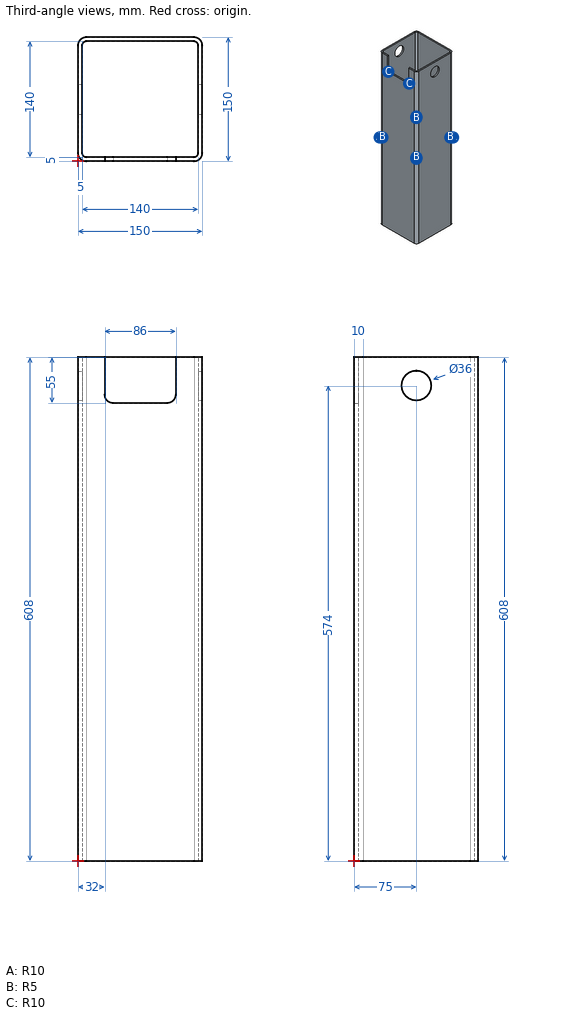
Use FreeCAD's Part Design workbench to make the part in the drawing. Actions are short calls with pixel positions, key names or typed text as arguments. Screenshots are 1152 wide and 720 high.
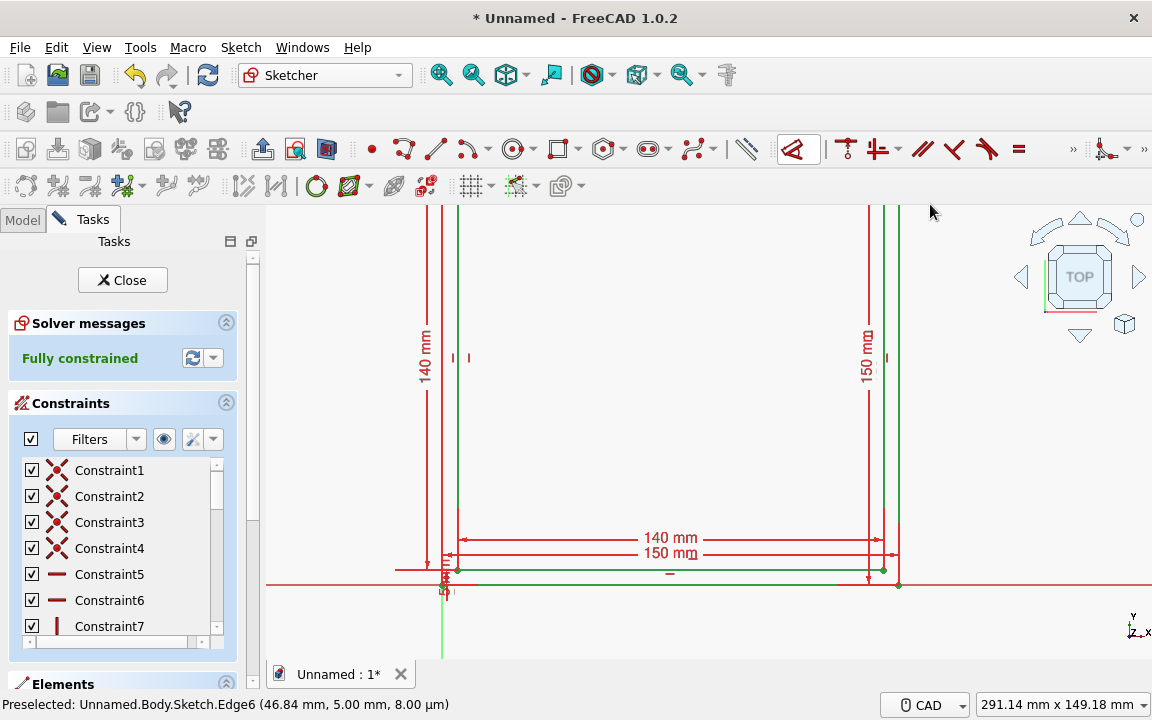
click(123, 280)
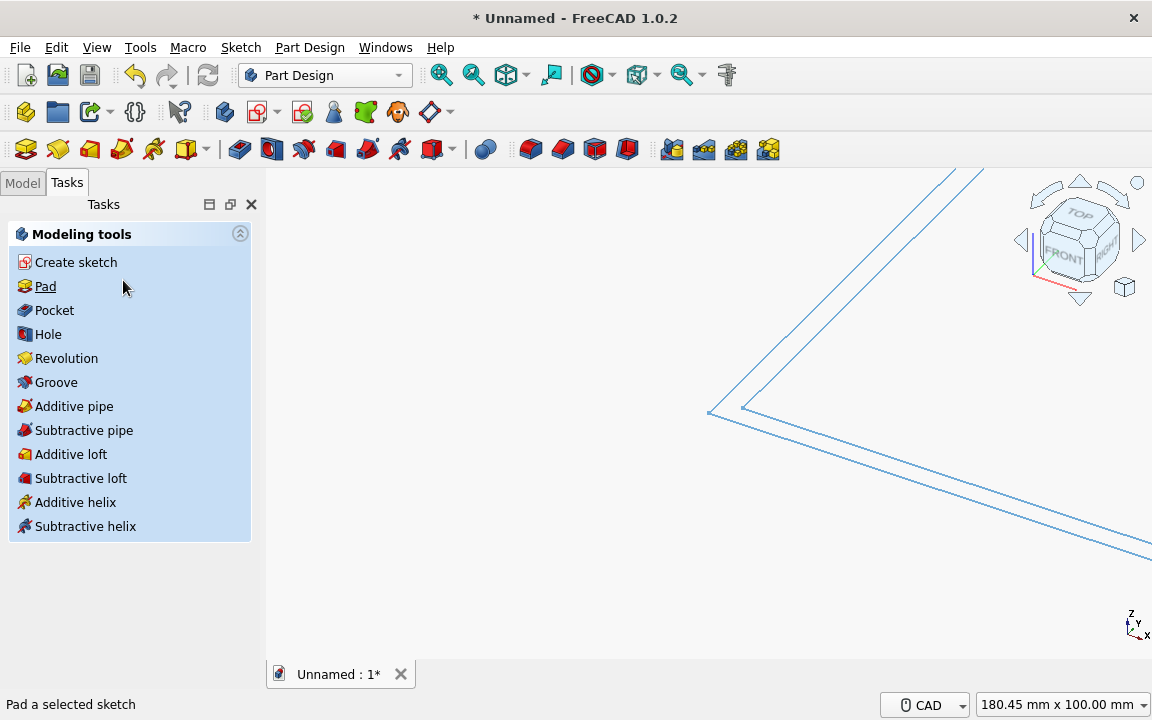
click(26, 150)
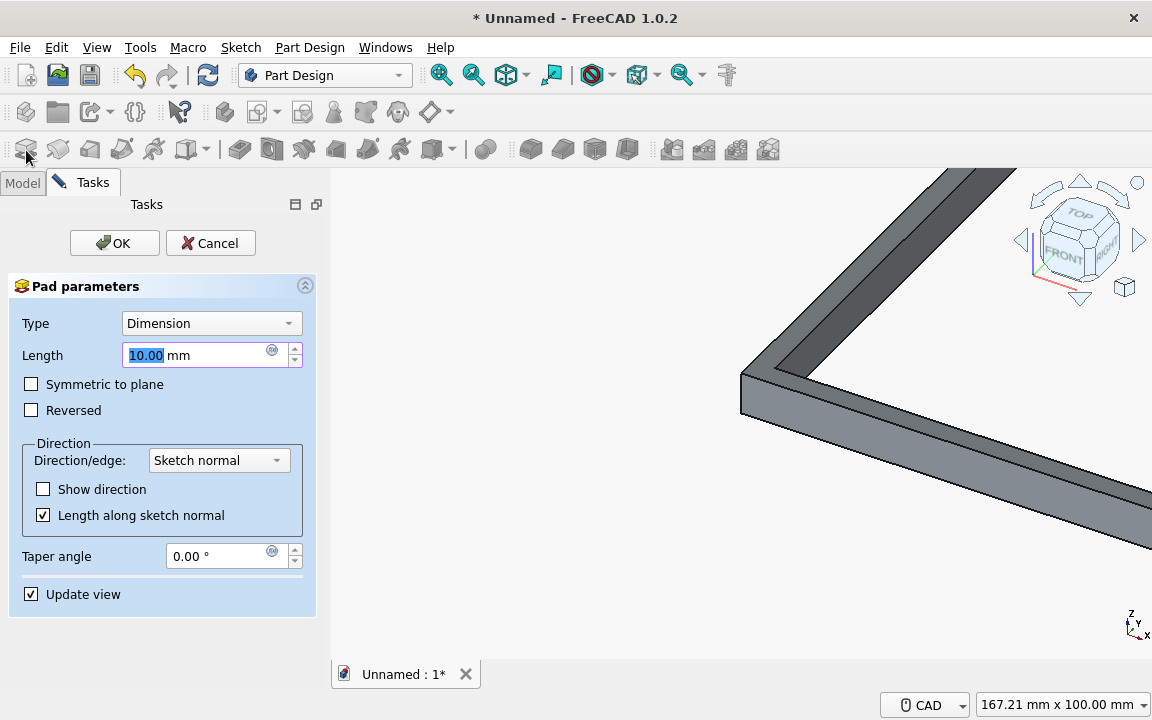
text(608)
key(Tab)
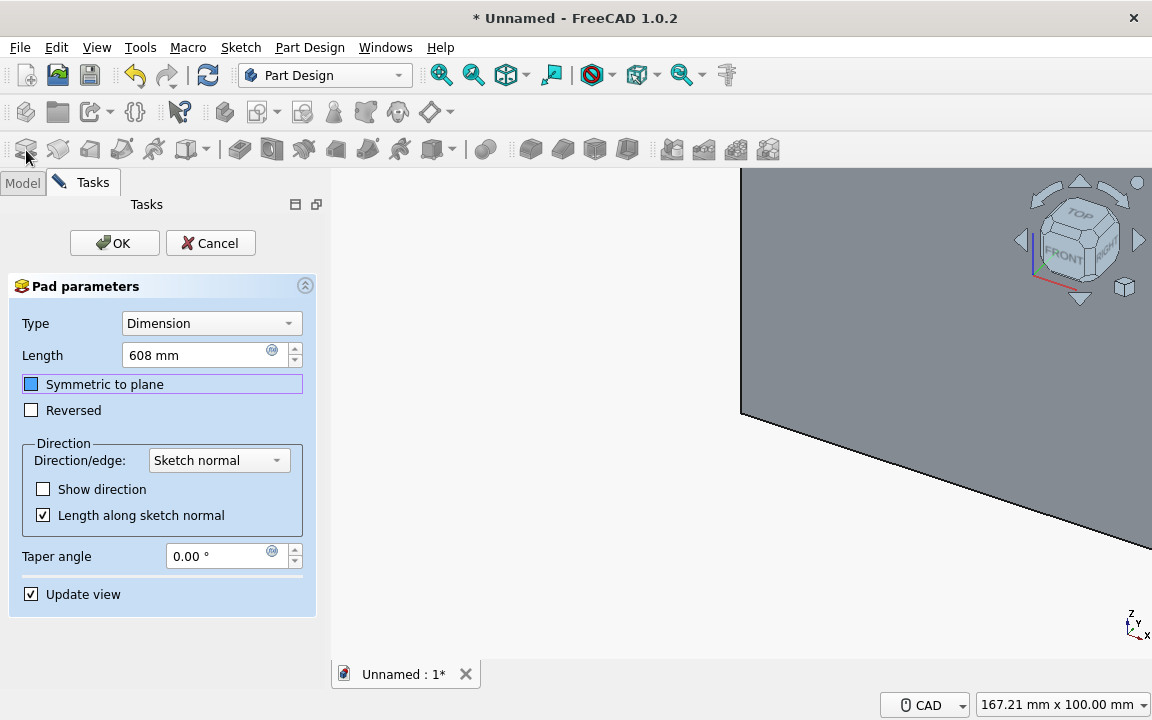
click(115, 243)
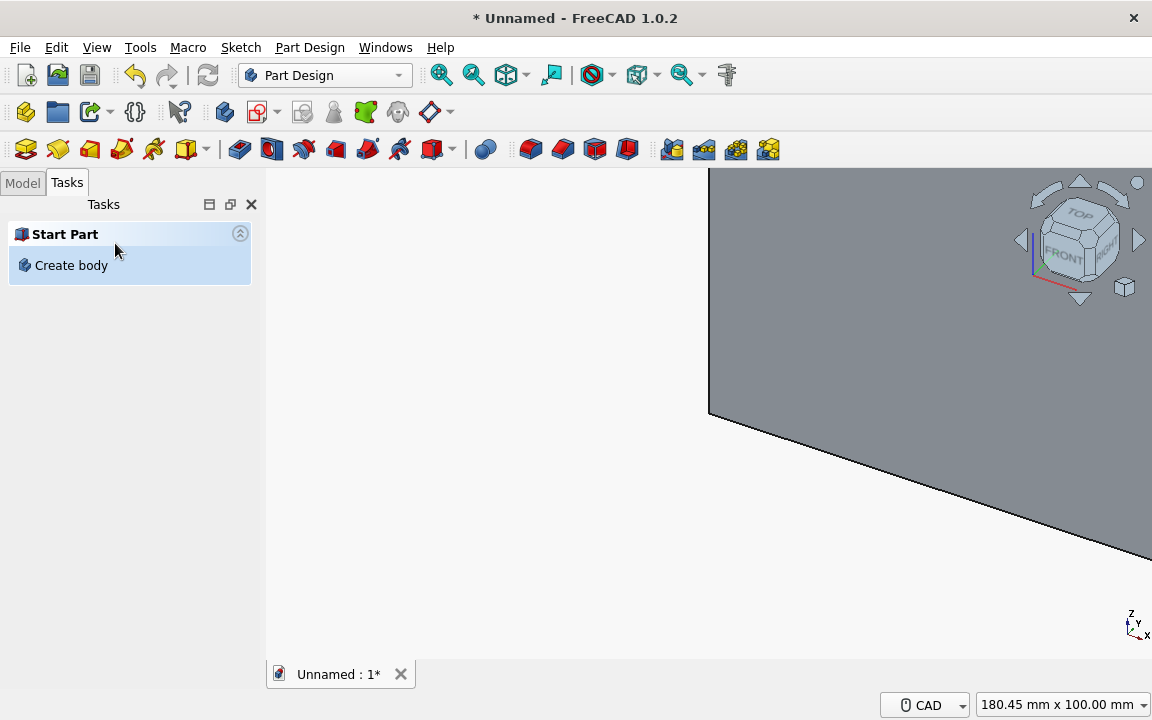
key(v)
key(f)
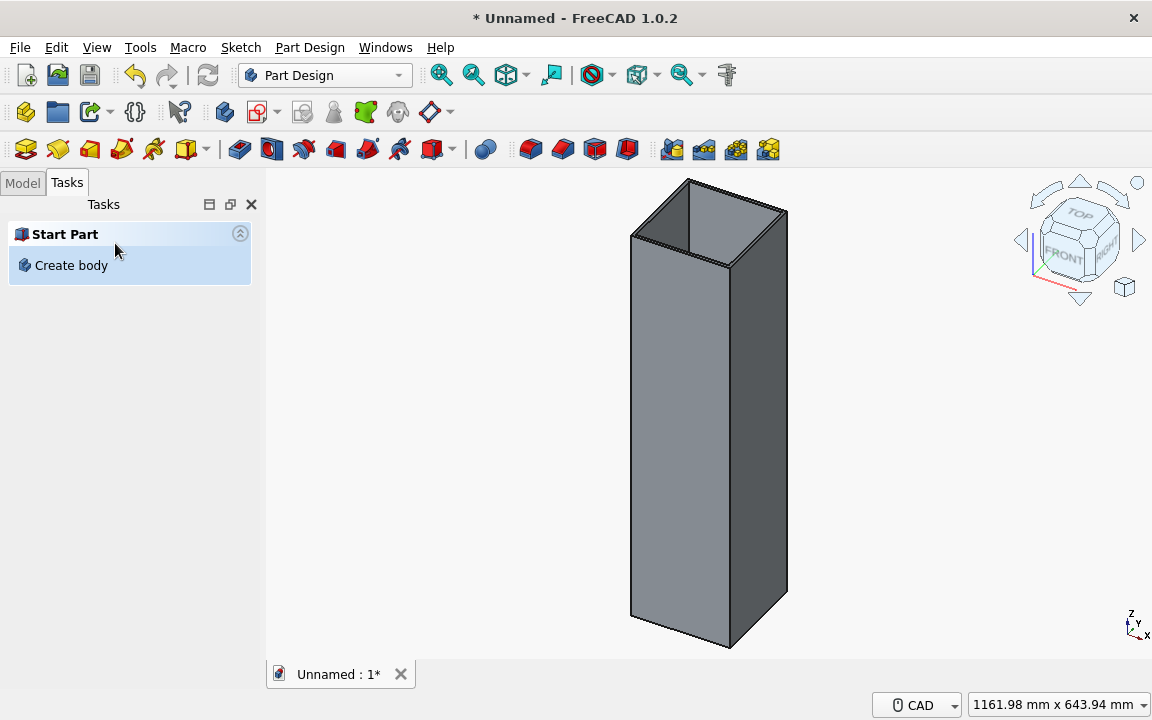
click(730, 457)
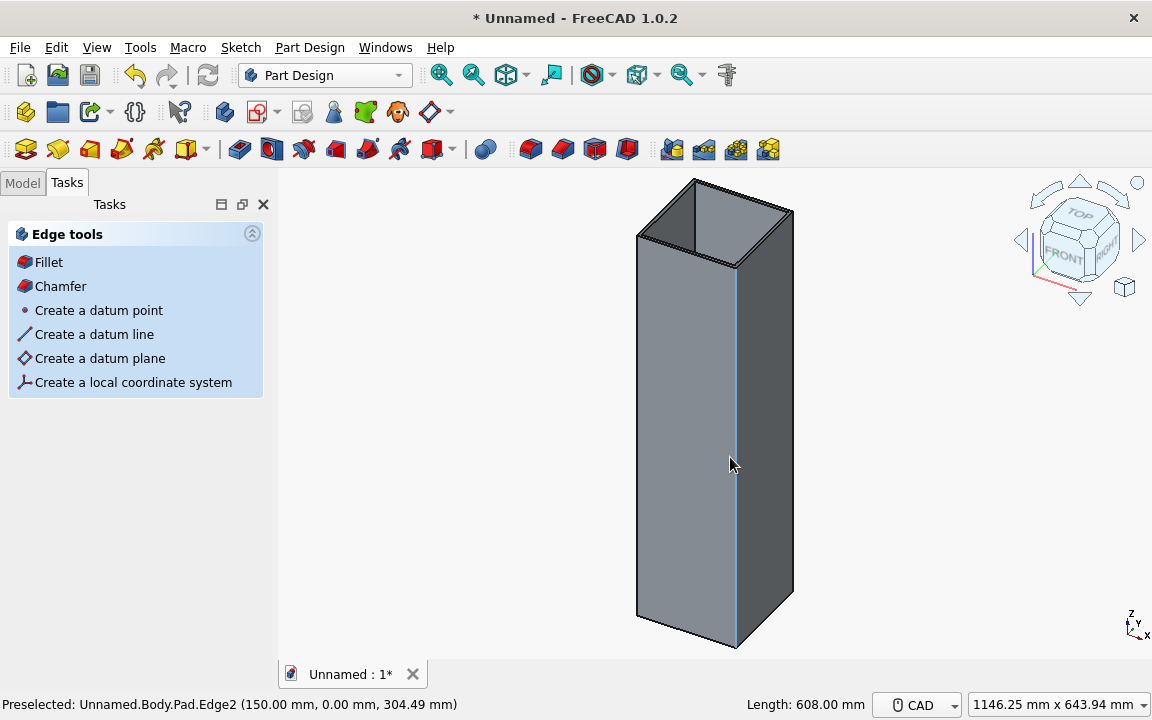
key(0)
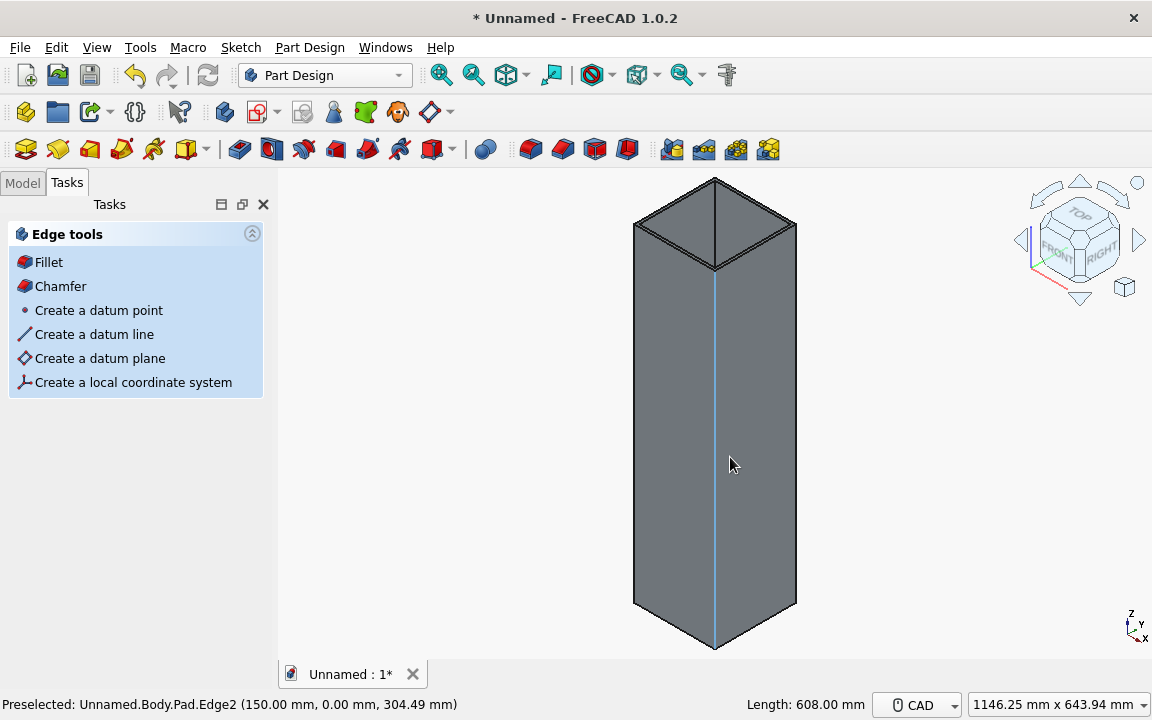
key(2)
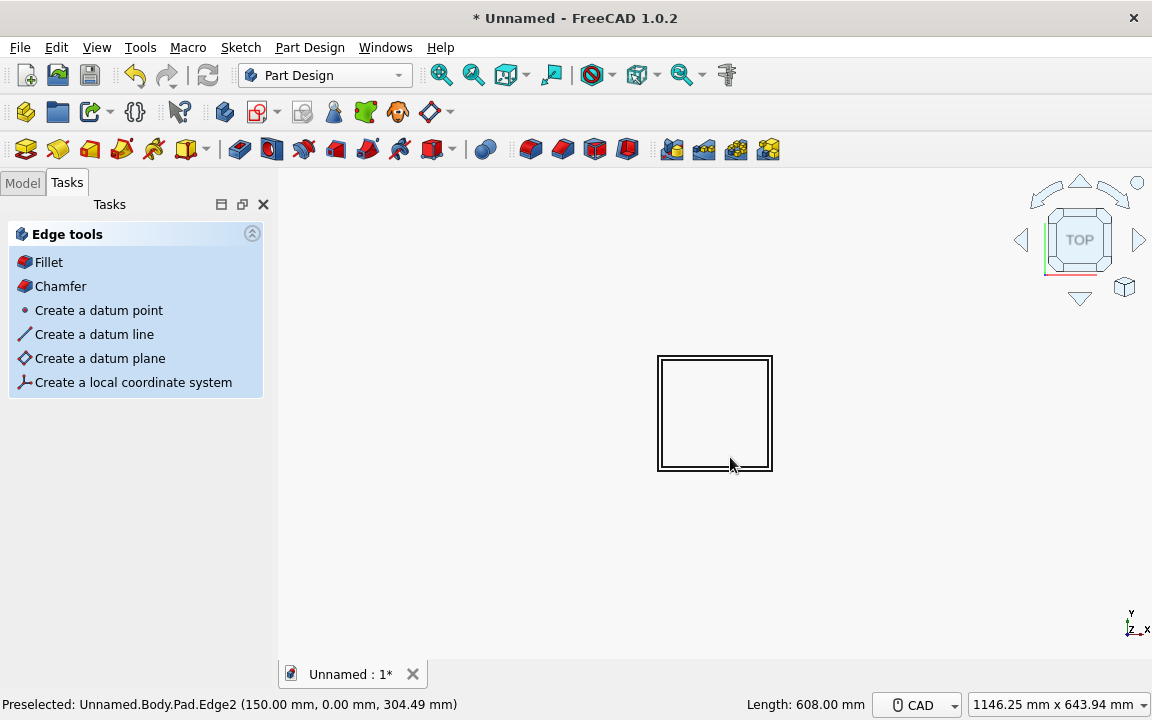
key(v)
key(f)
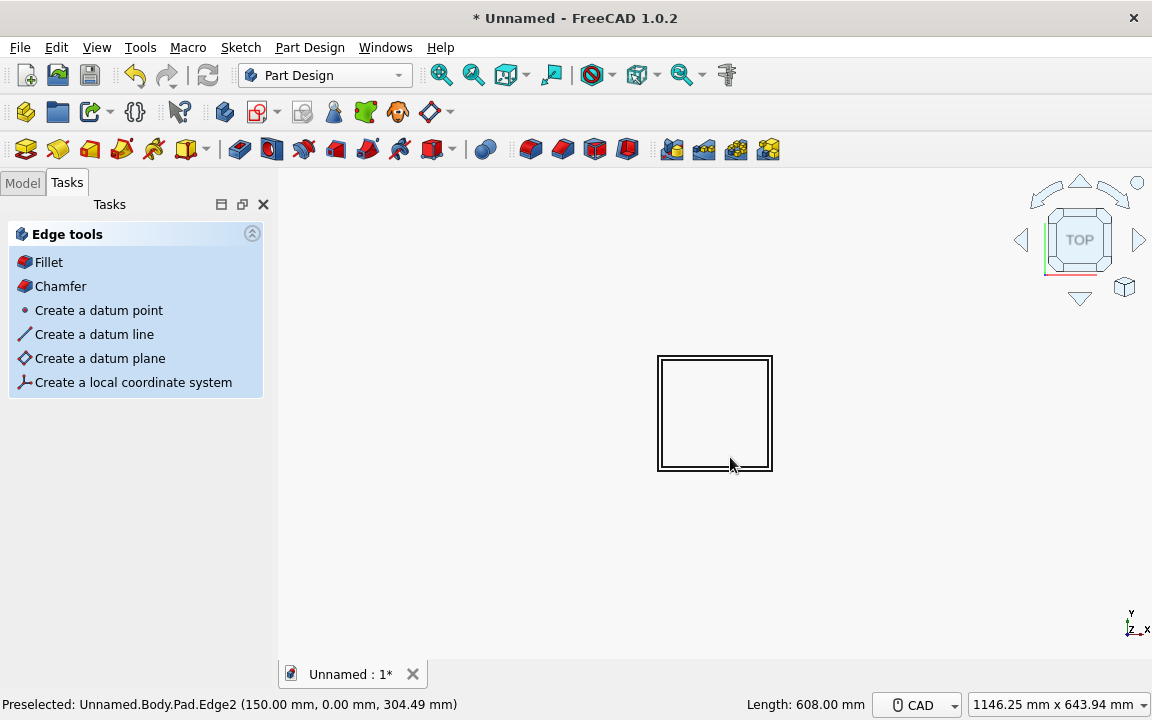
key(1)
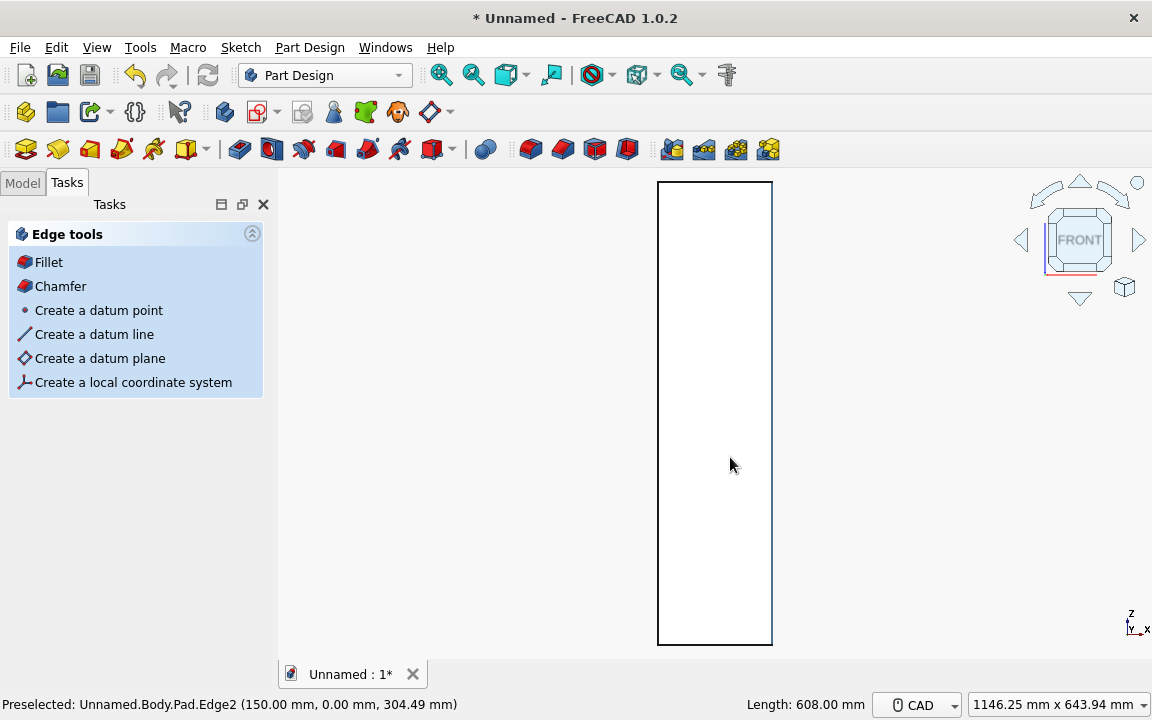
key(3)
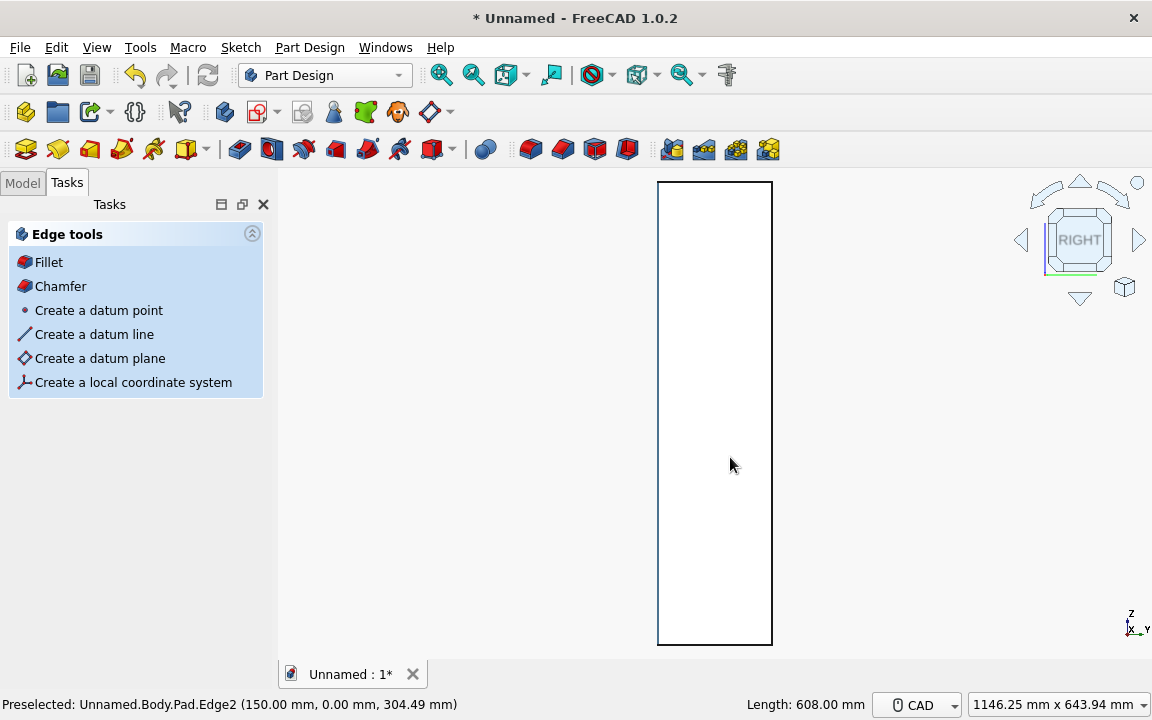
click(772, 412, ctrl)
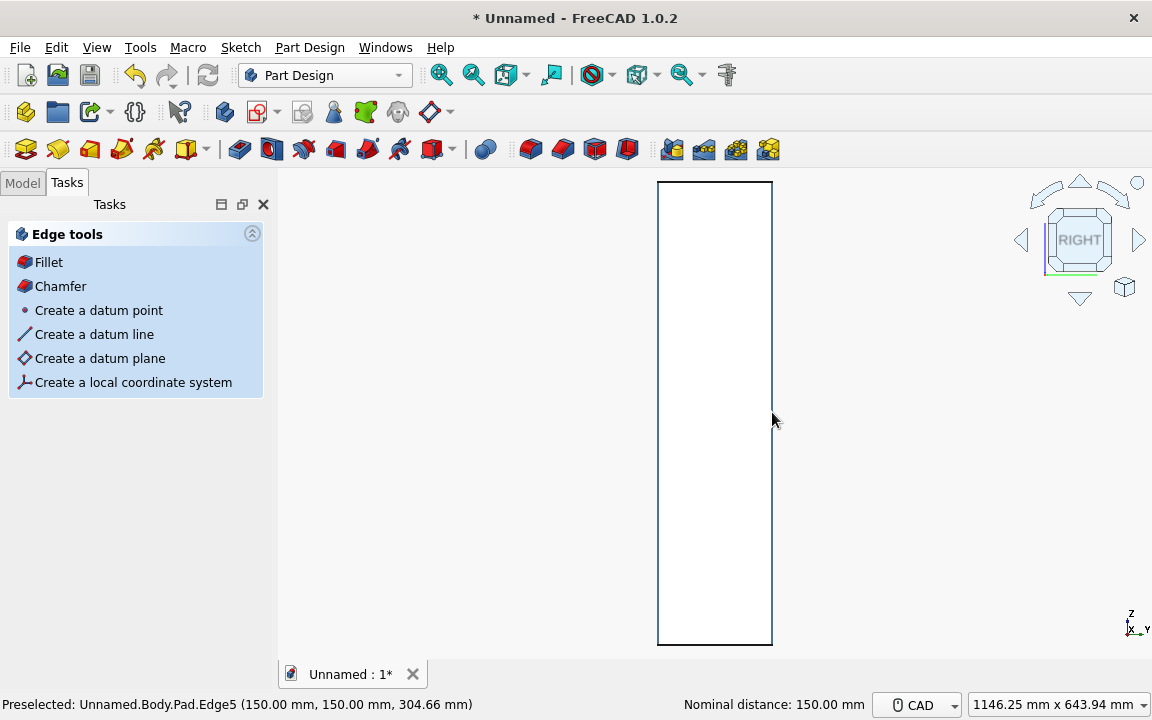
key(5)